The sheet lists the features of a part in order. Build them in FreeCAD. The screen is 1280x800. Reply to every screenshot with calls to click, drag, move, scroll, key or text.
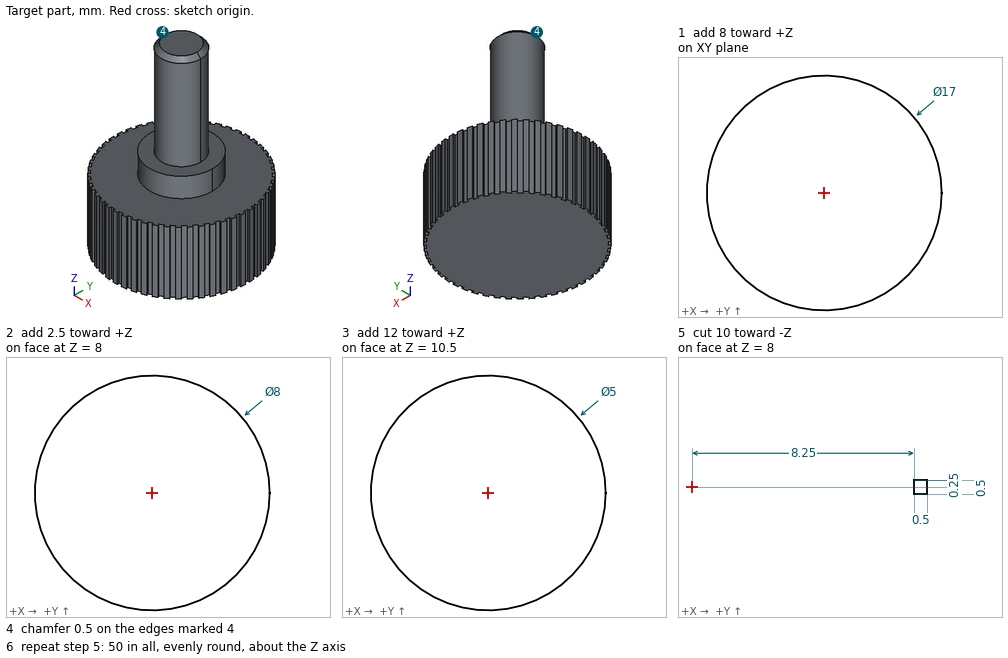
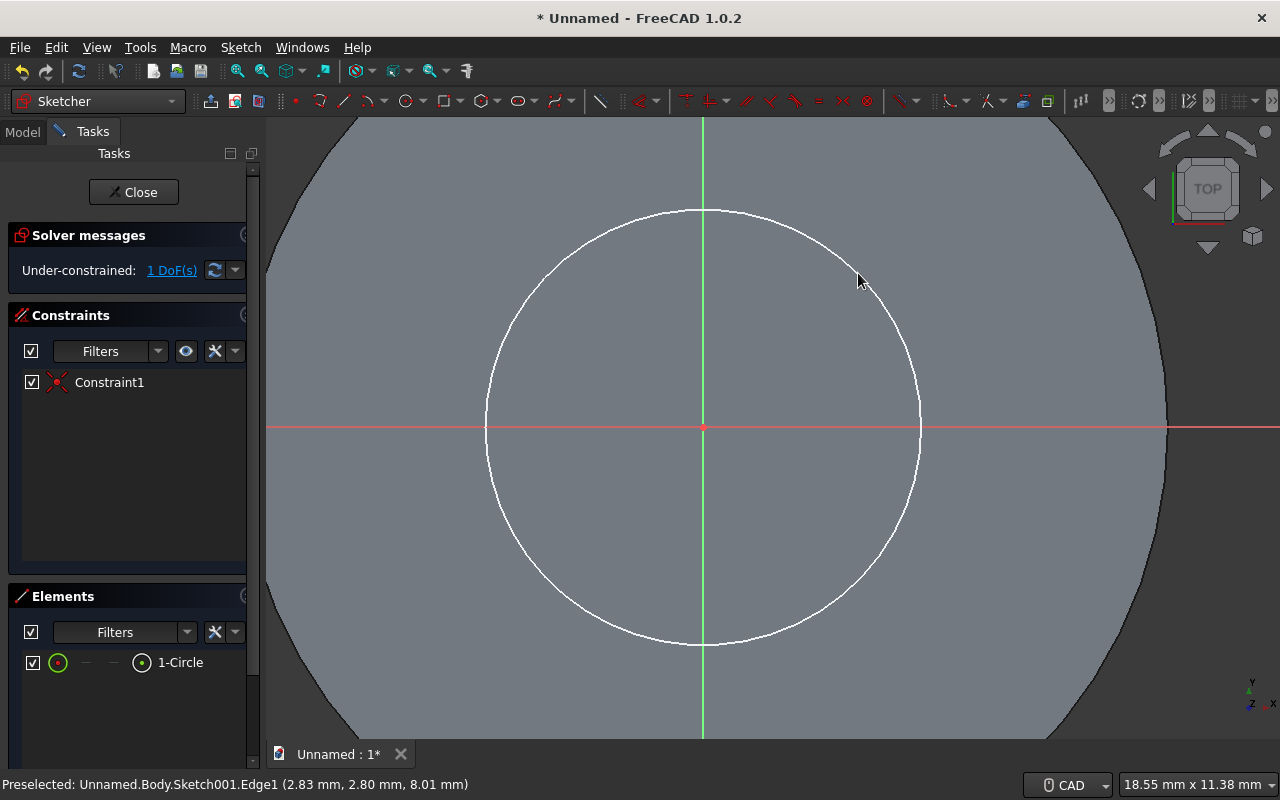
click(640, 102)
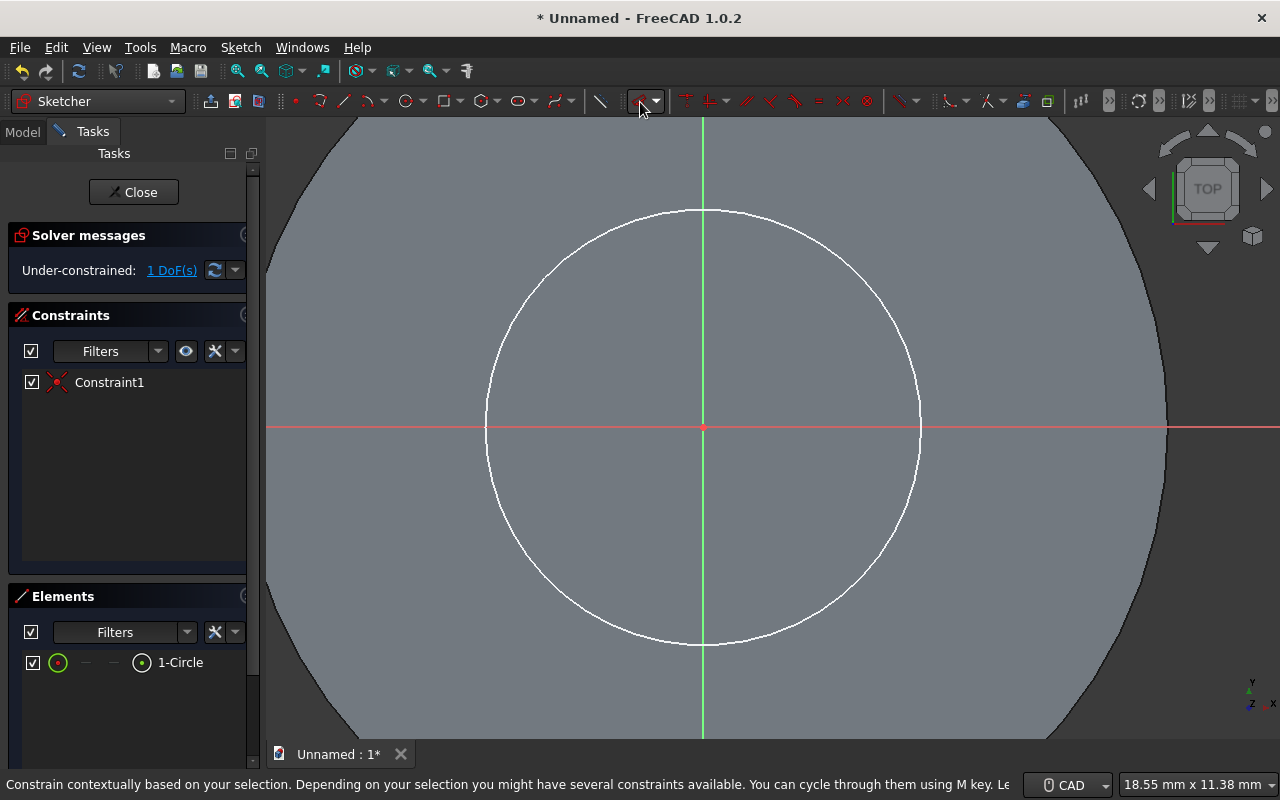
click(857, 273)
click(880, 250)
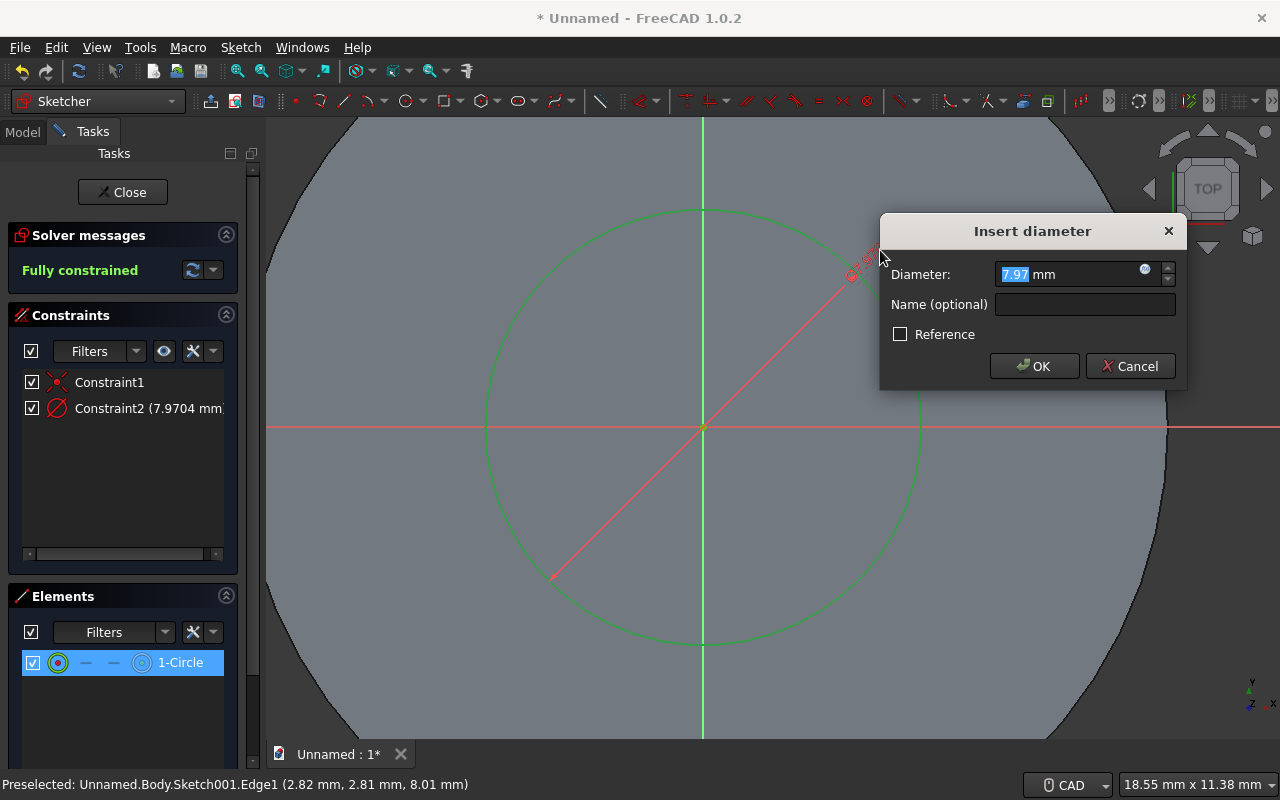
text(8)
key(Return)
key(Escape)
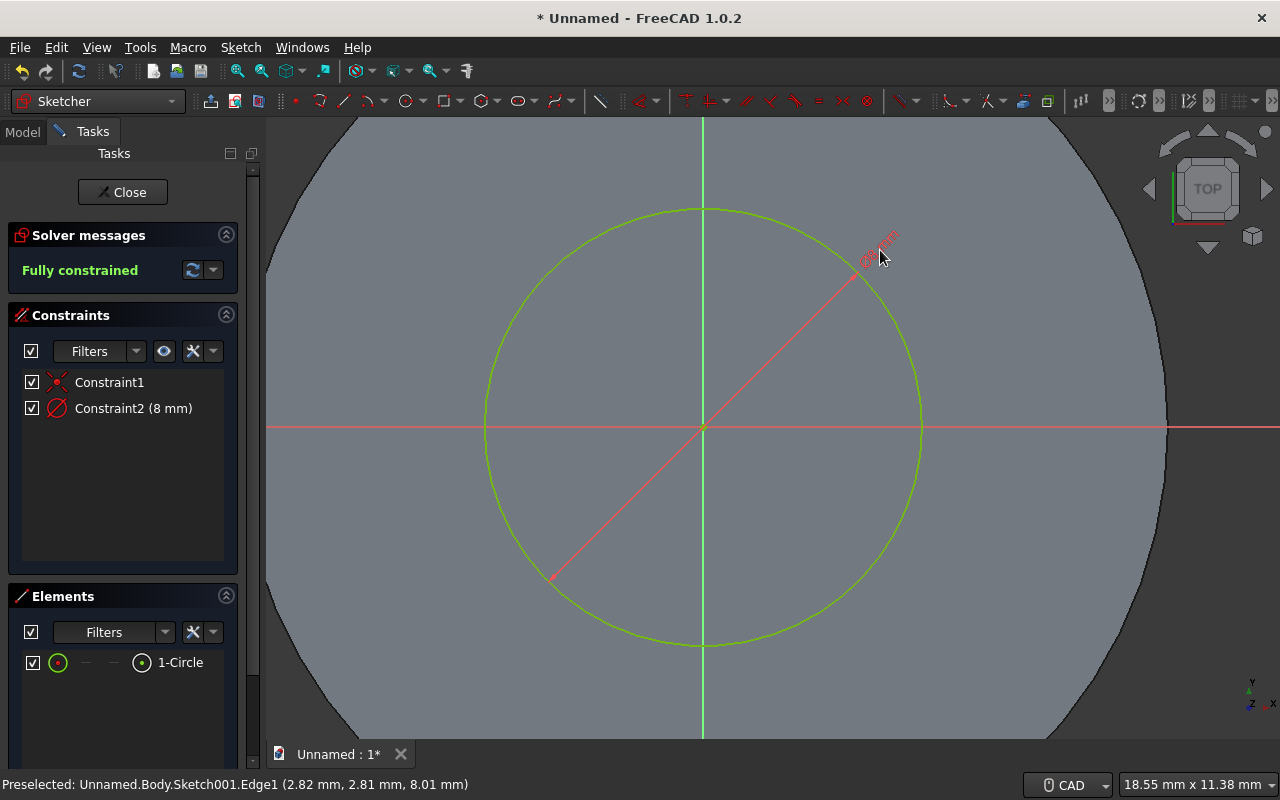
click(123, 192)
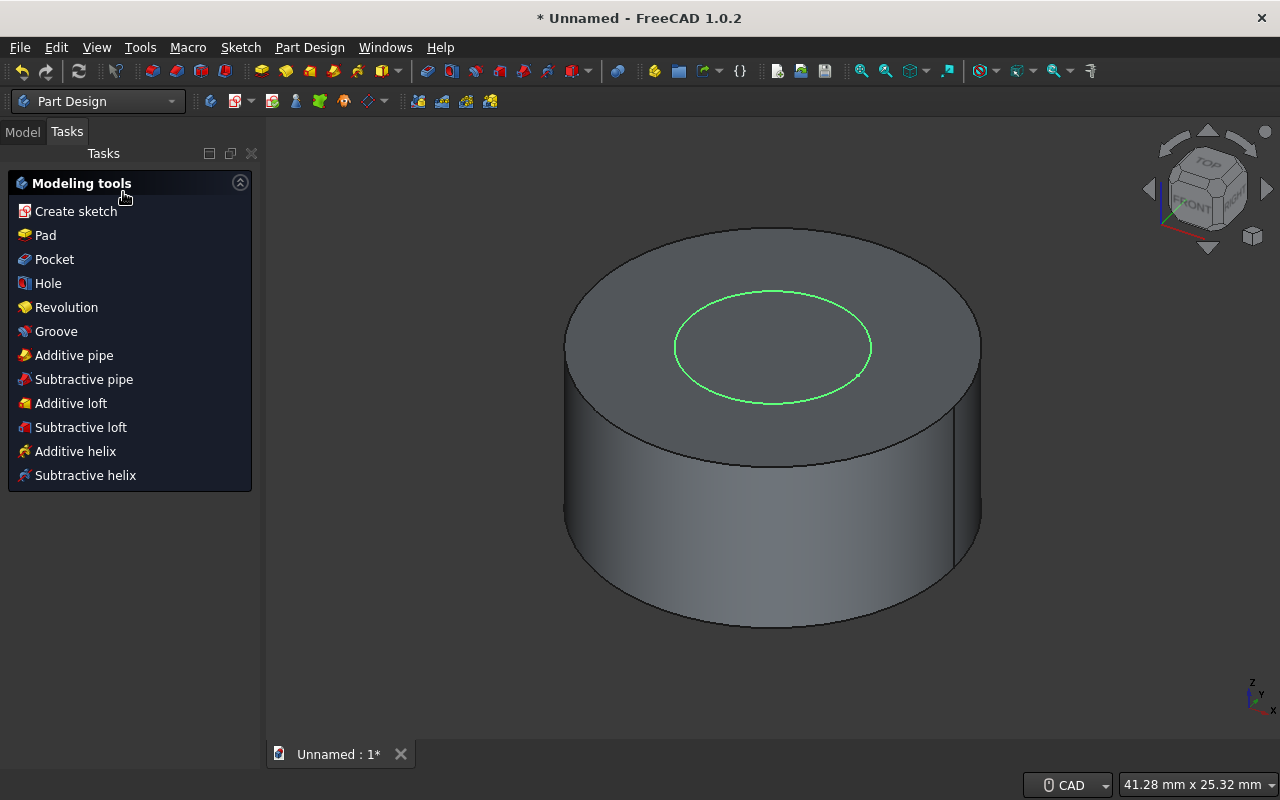
click(262, 72)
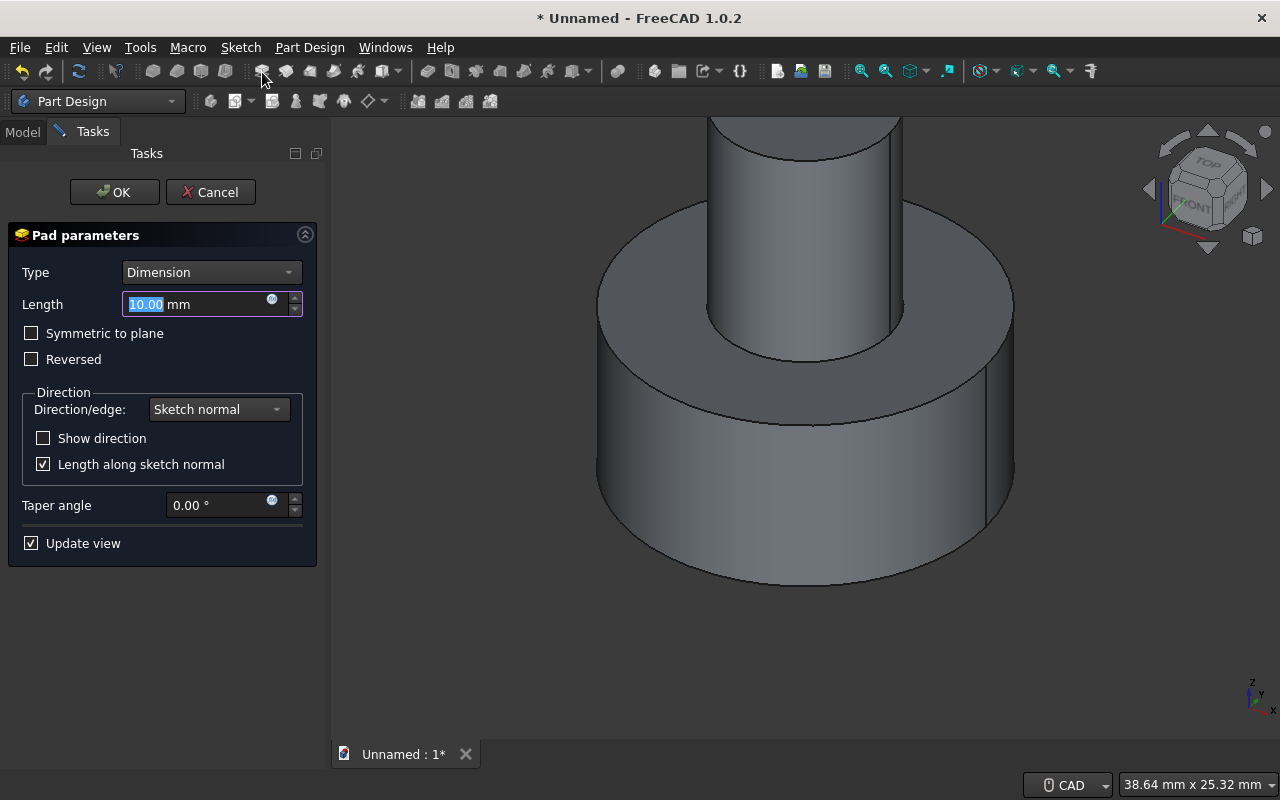
text(2.5)
key(Tab)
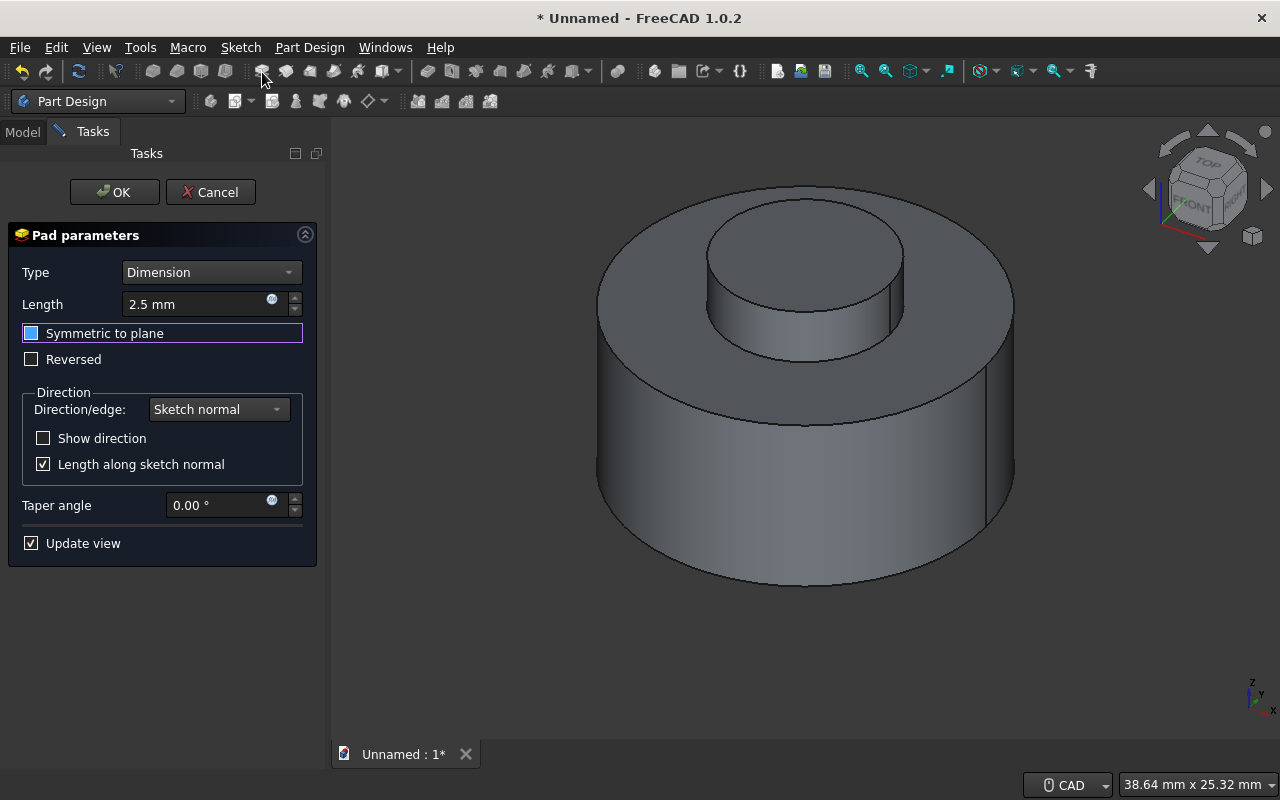
click(115, 192)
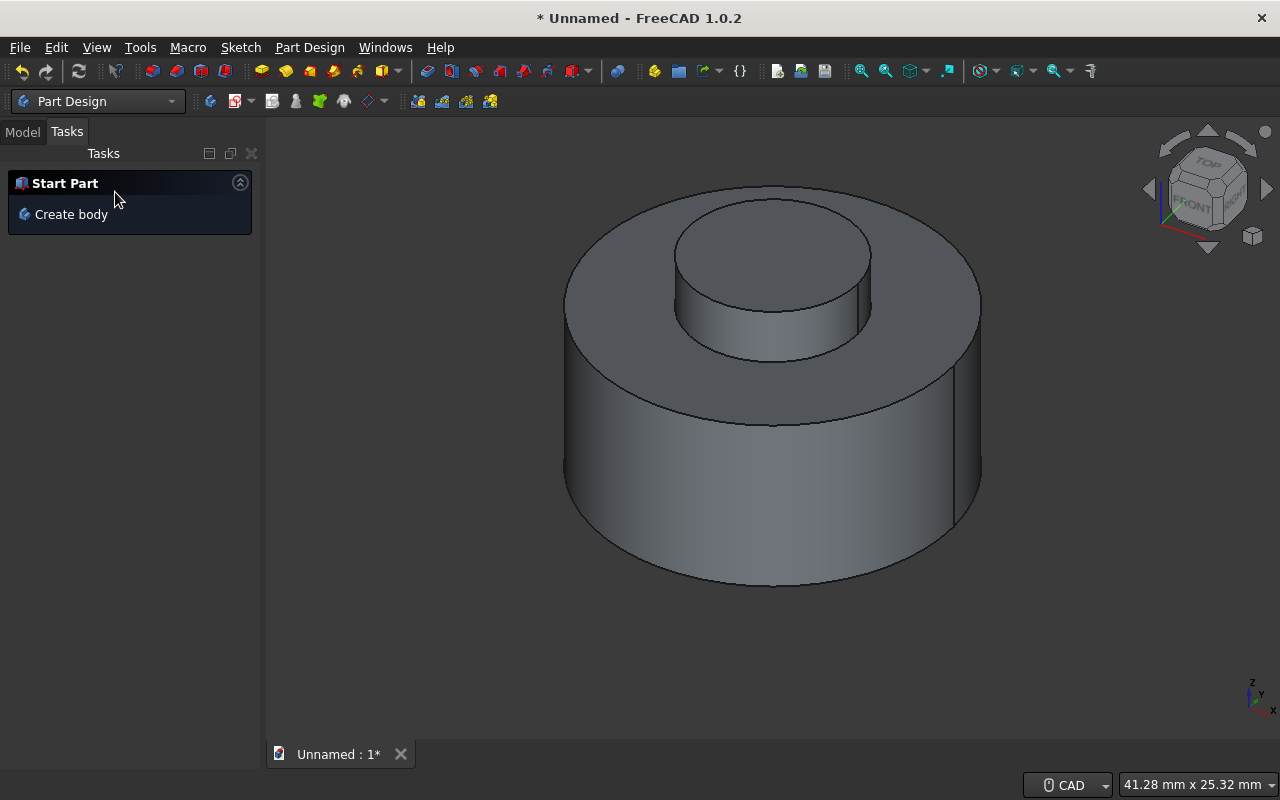
key(v)
key(f)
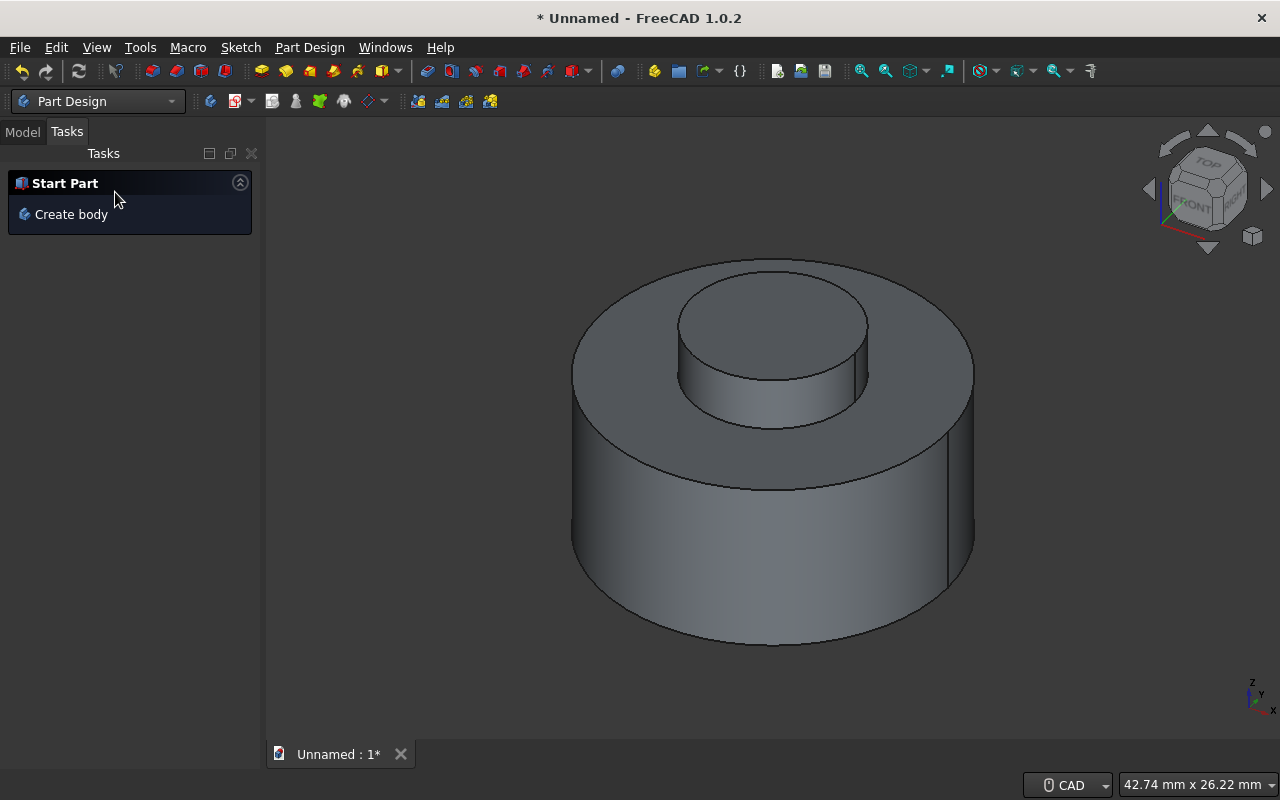
click(773, 325)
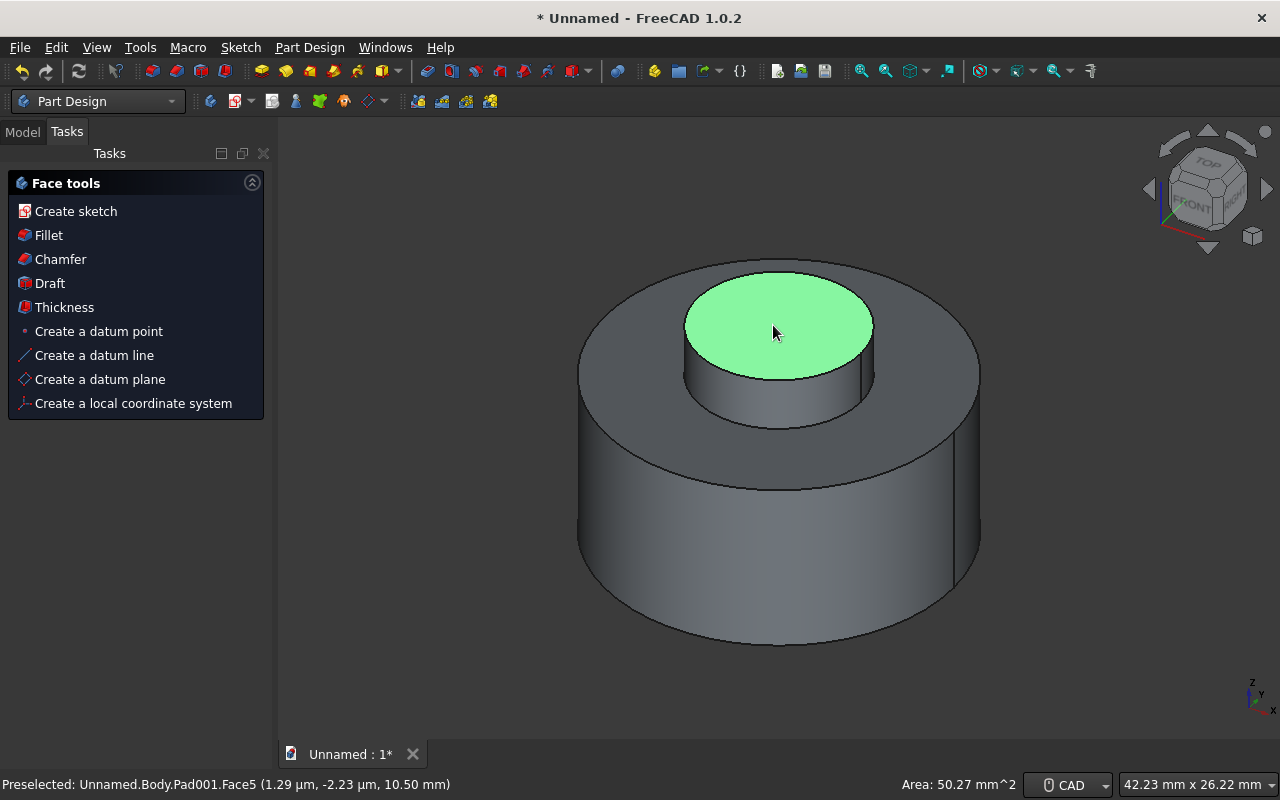
click(236, 102)